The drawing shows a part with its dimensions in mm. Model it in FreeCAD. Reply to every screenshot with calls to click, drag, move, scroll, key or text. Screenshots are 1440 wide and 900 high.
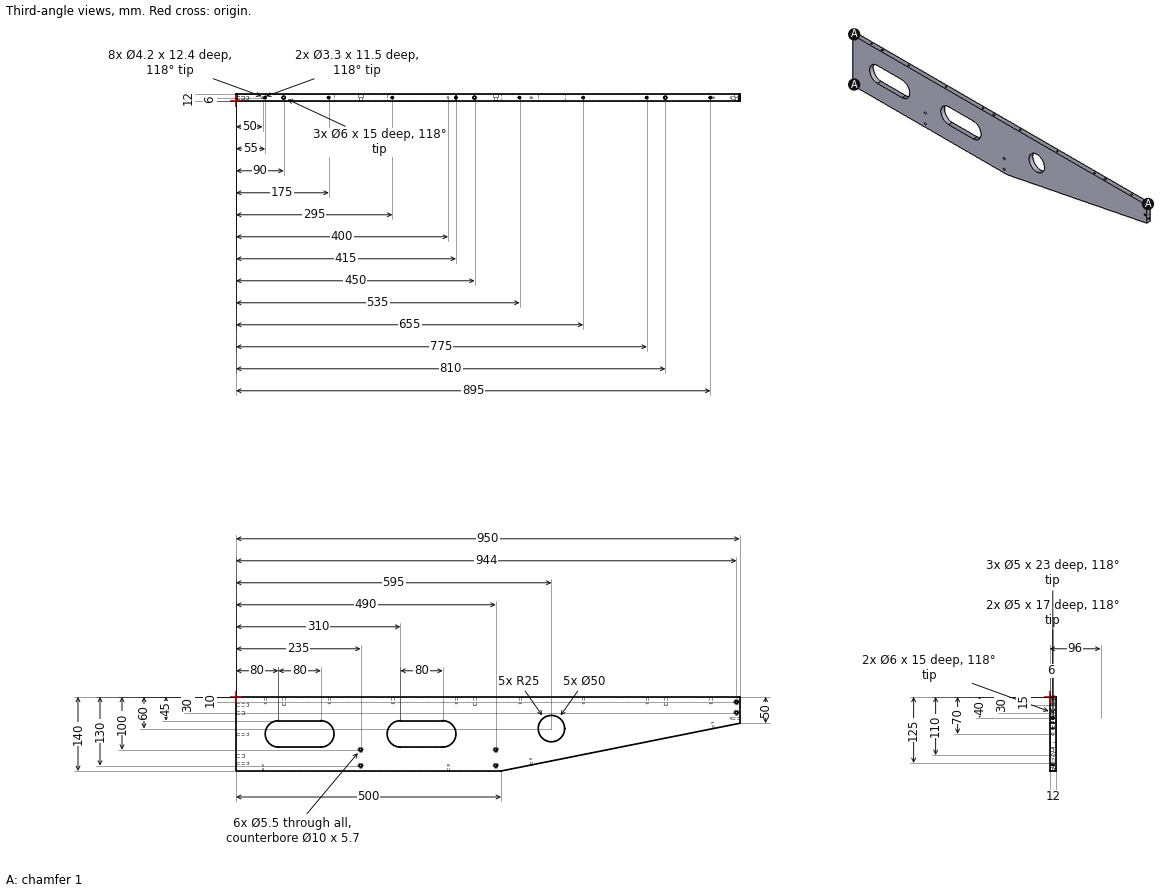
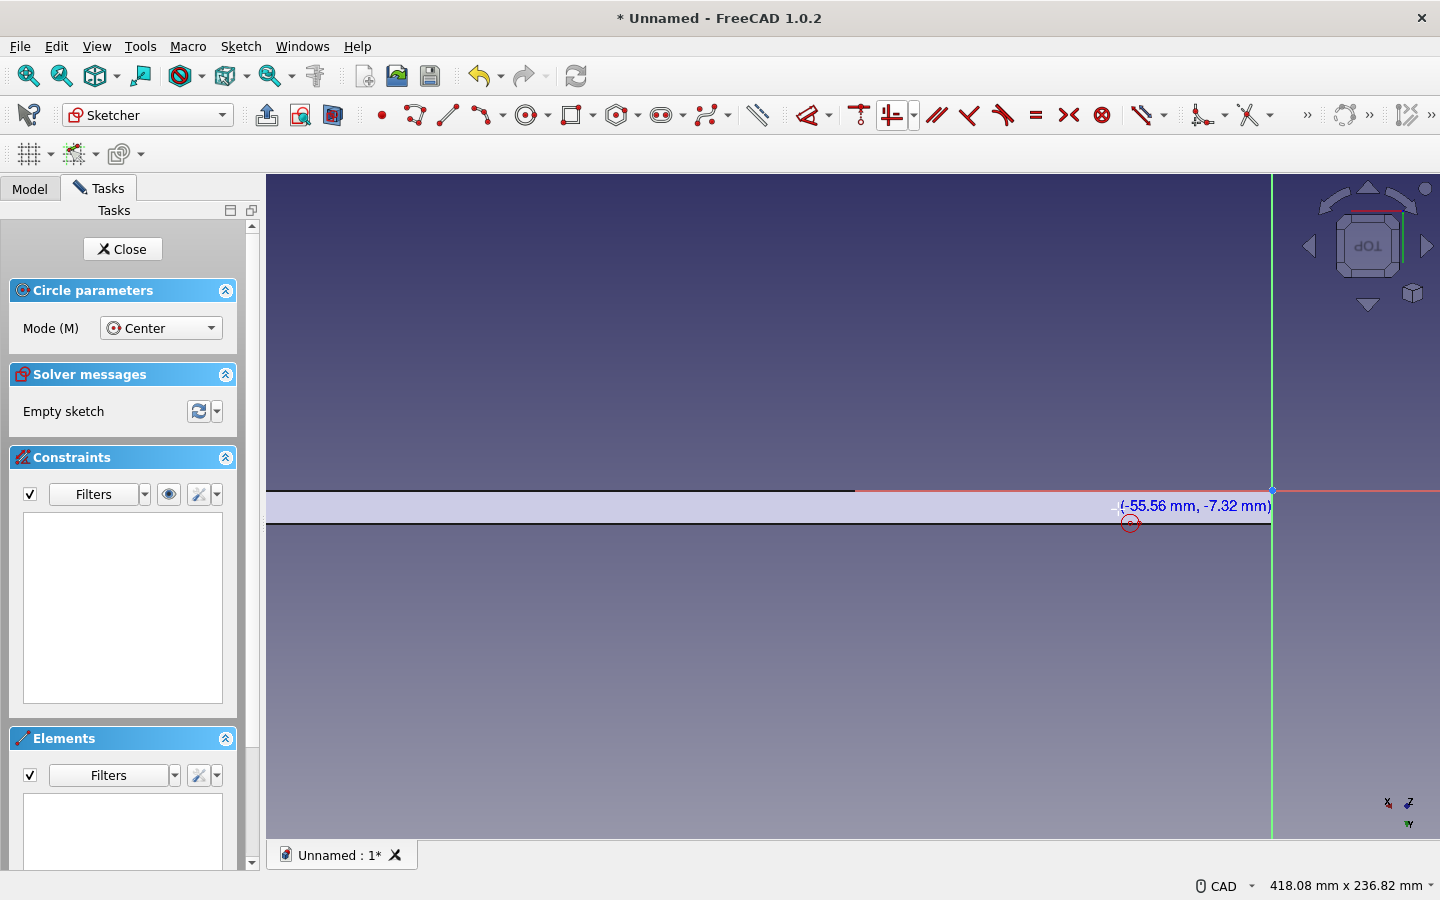
click(1118, 507)
move(1122, 512)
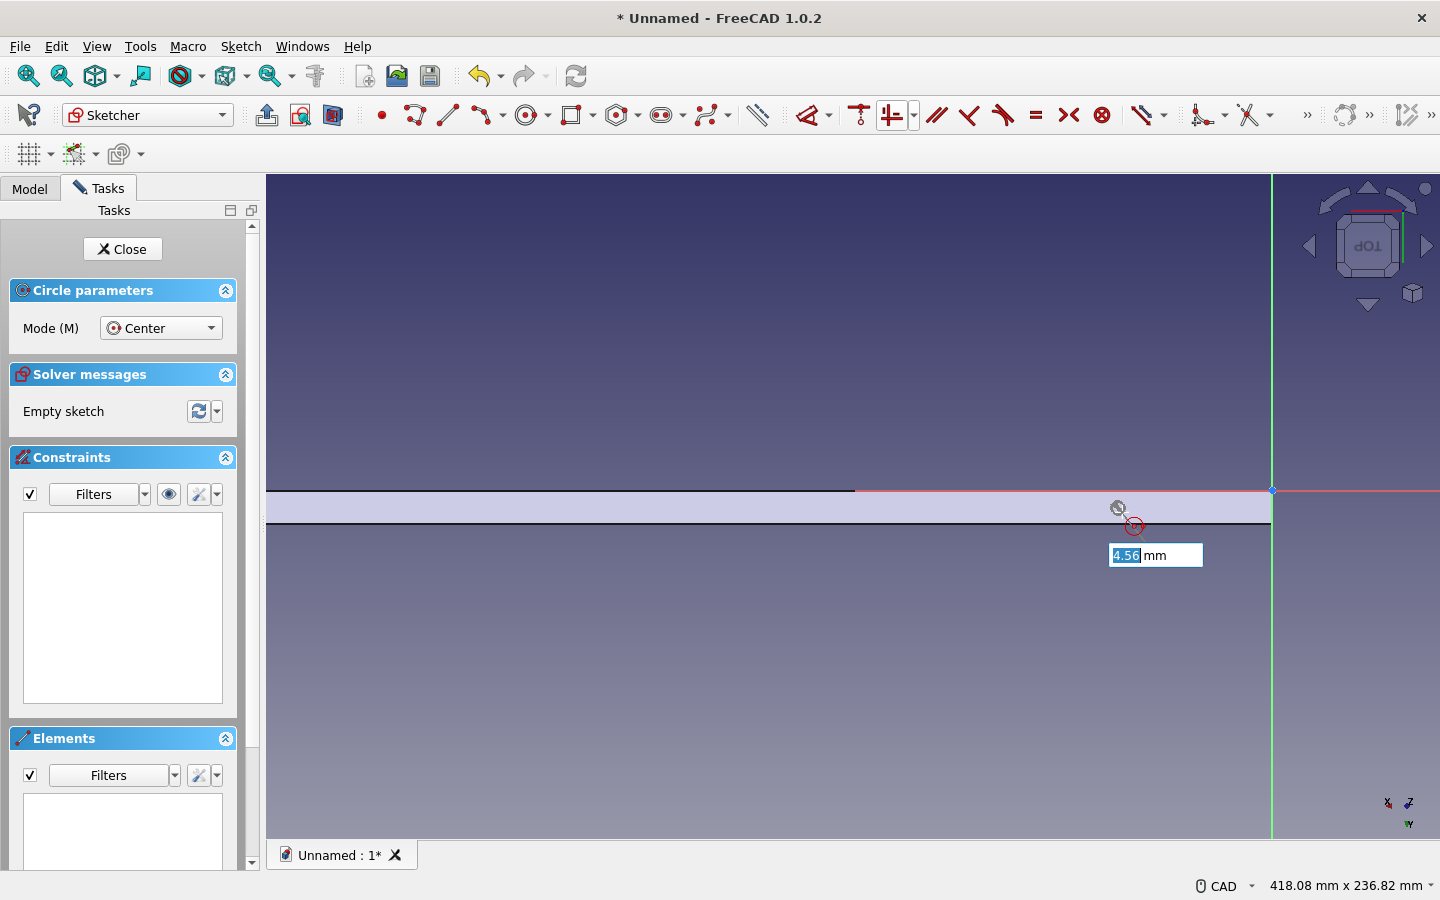
text(4.2)
key(Return)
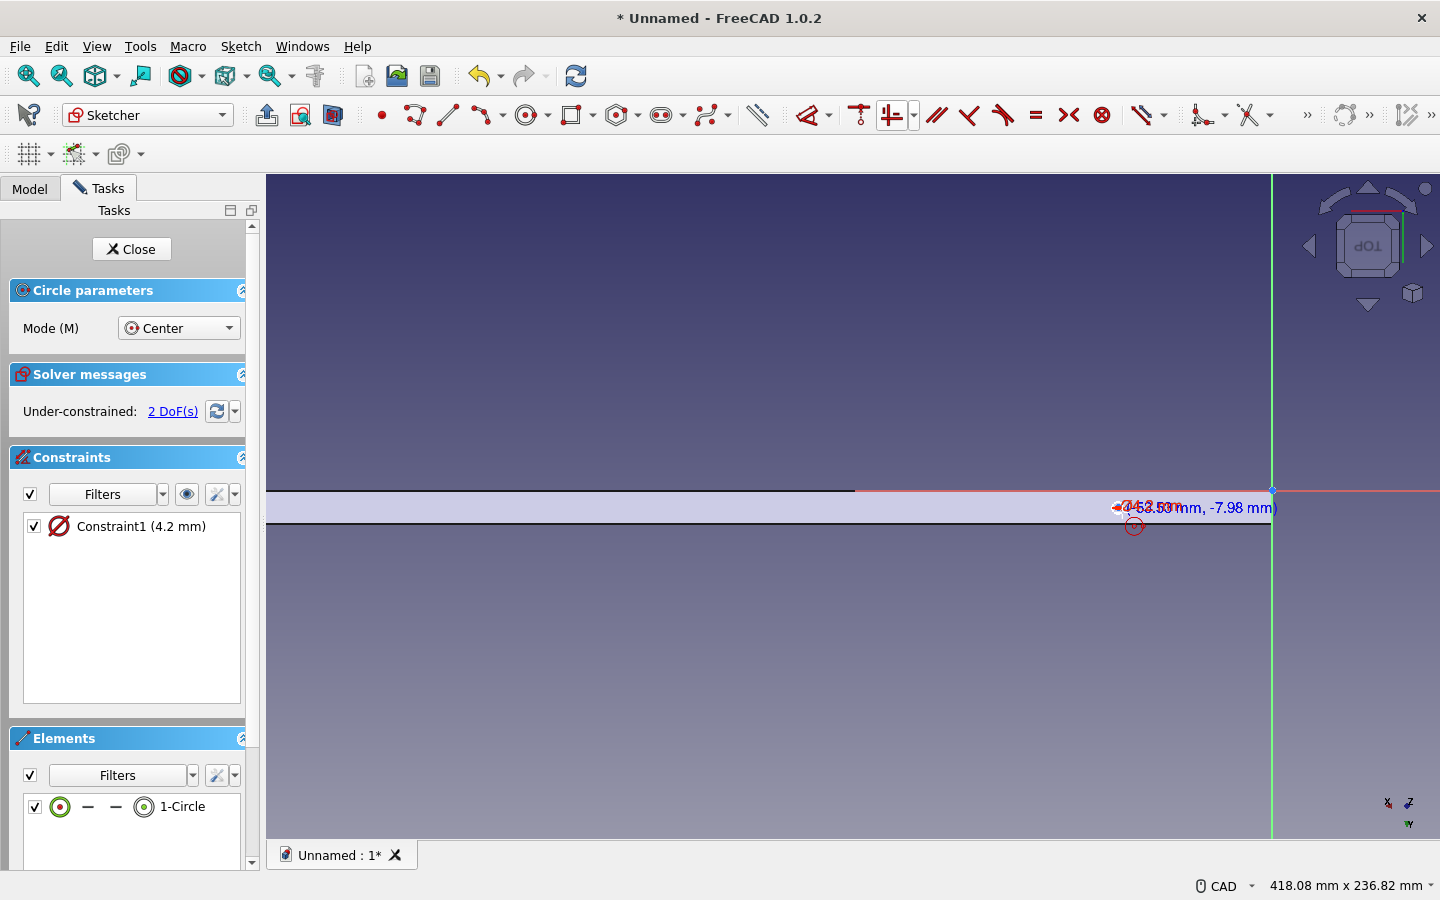
scroll(781, 507, up, 7)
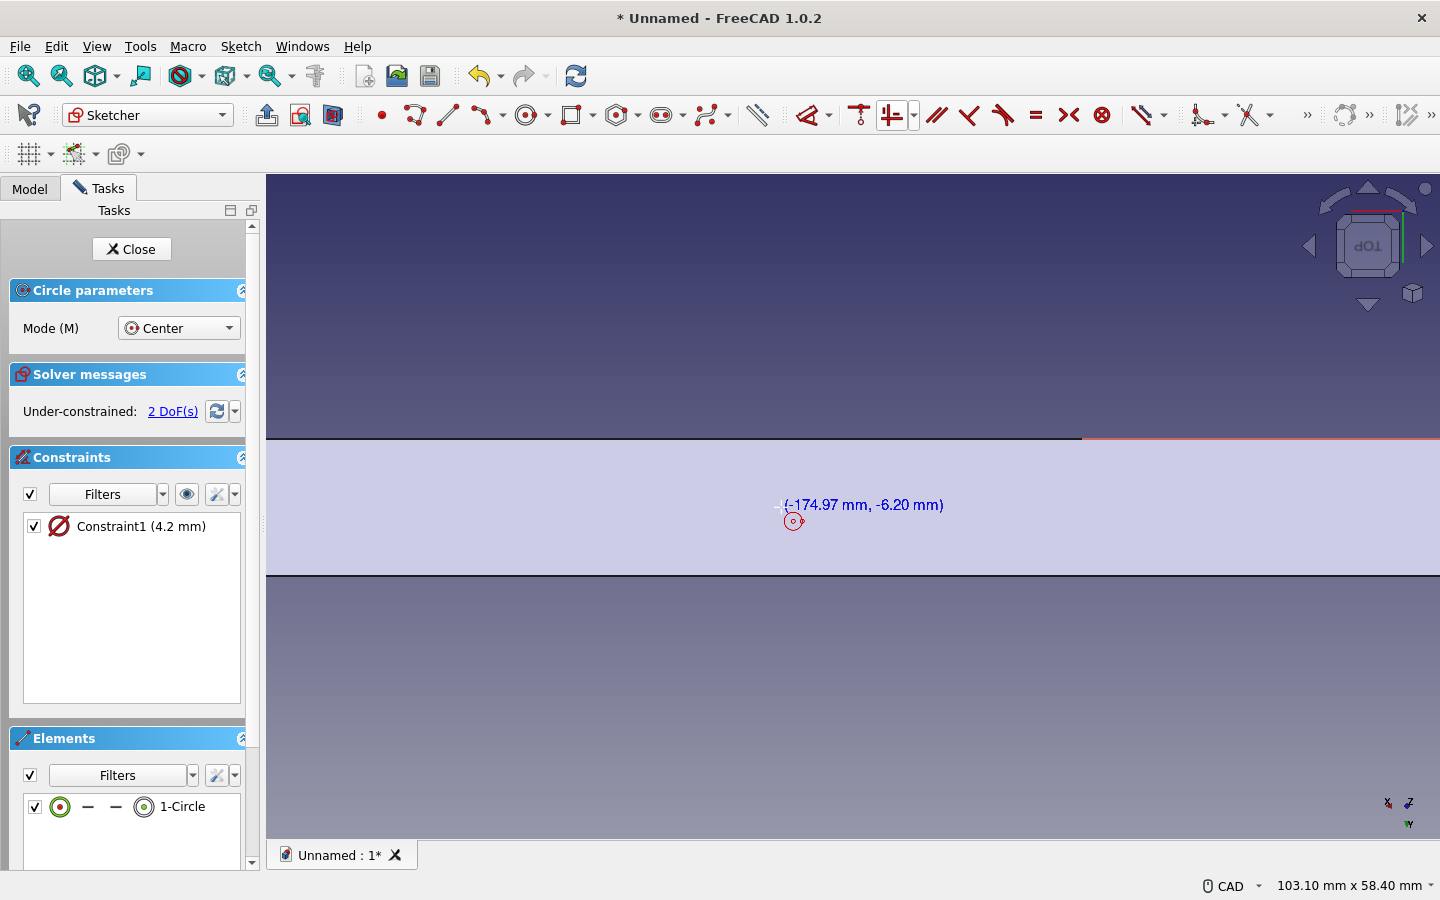
scroll(1035, 508, down, 13)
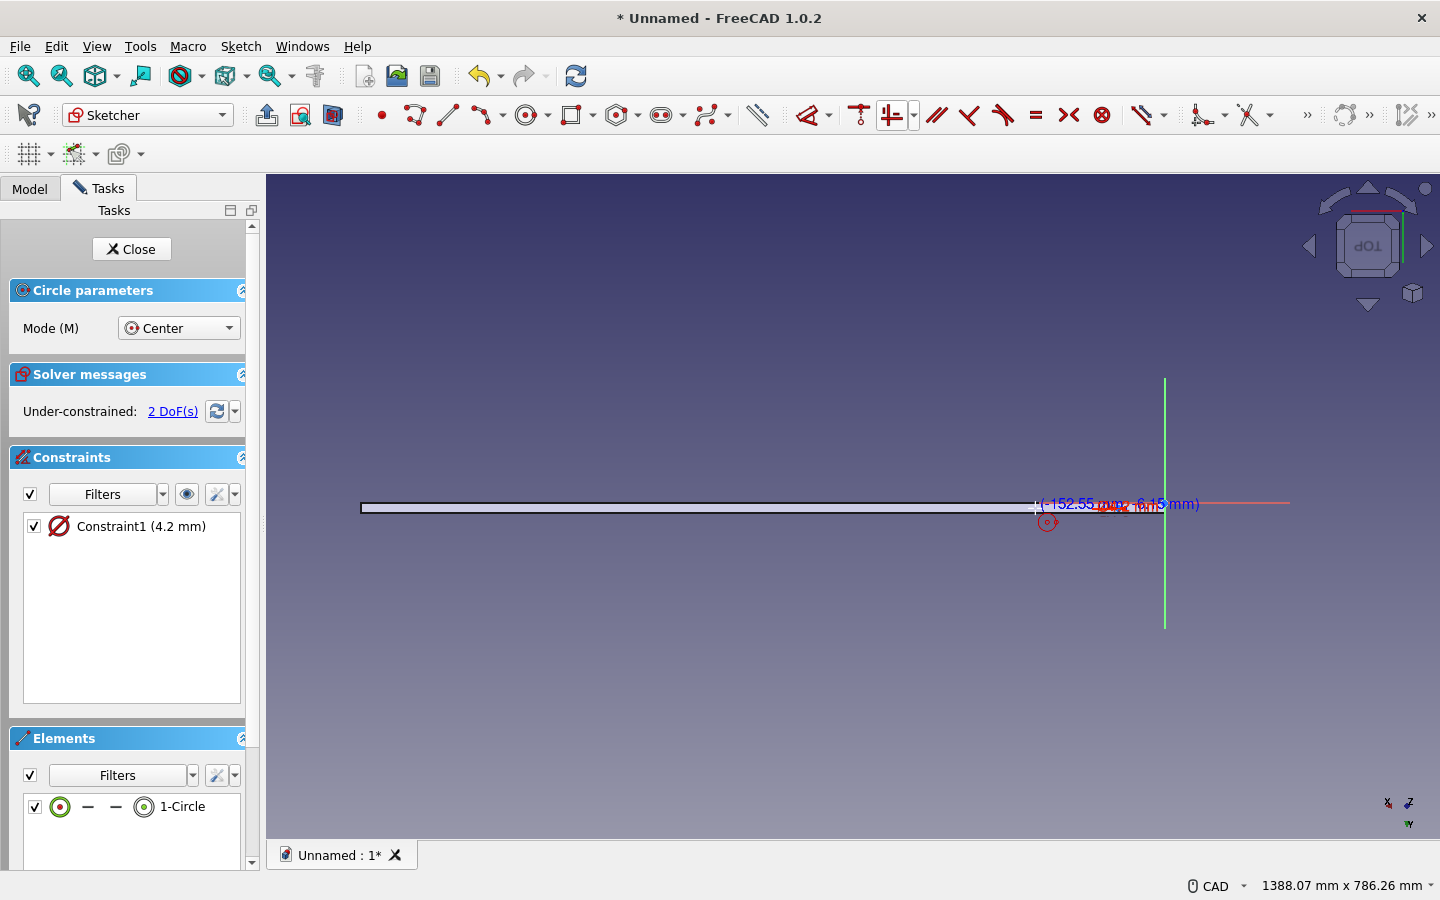
scroll(1017, 508, up, 6)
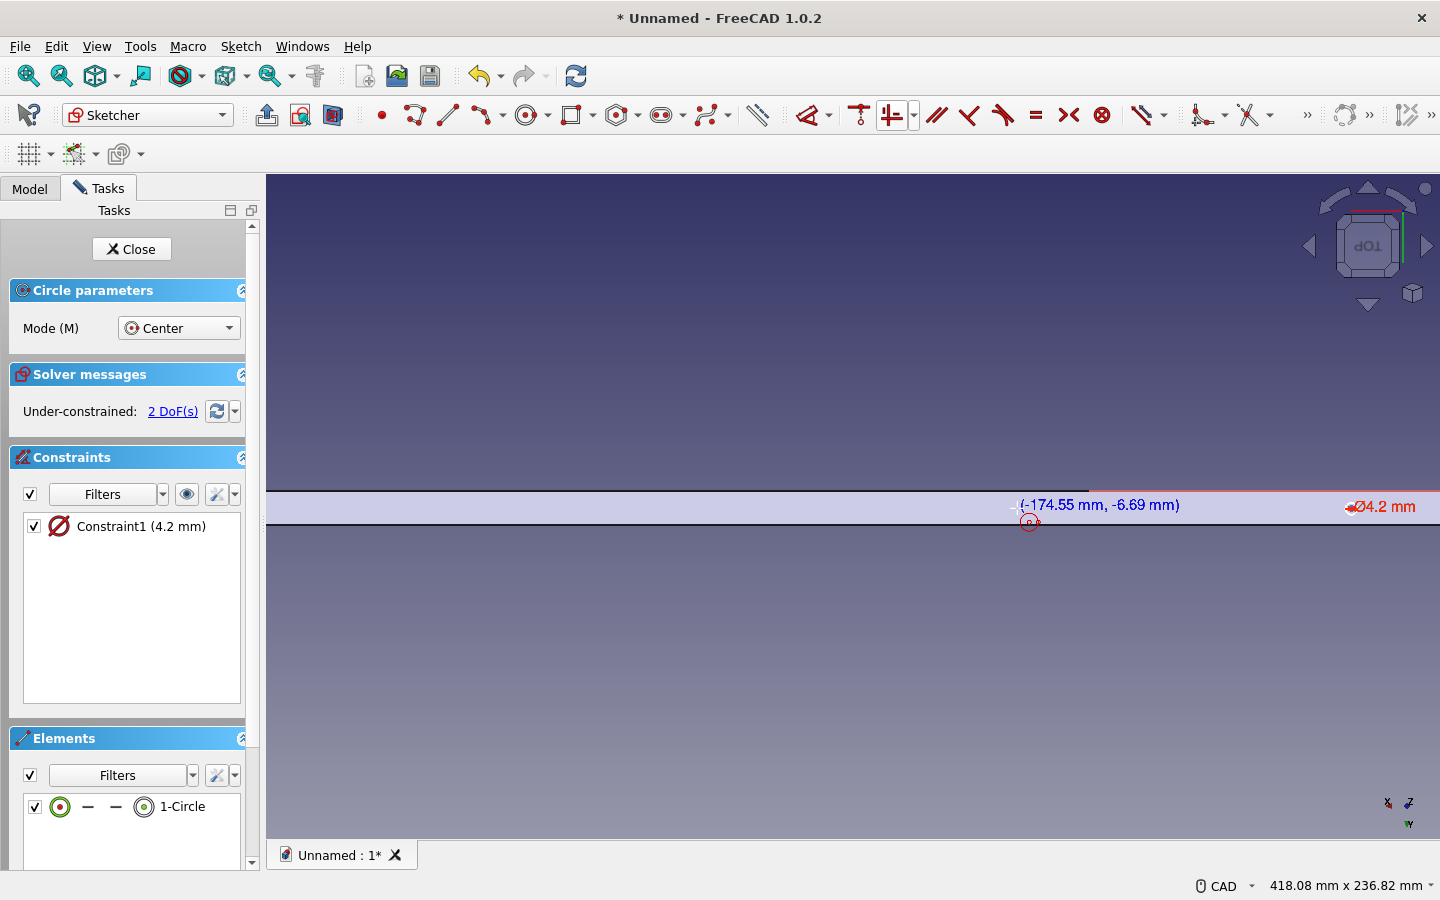
click(1014, 508)
move(1018, 512)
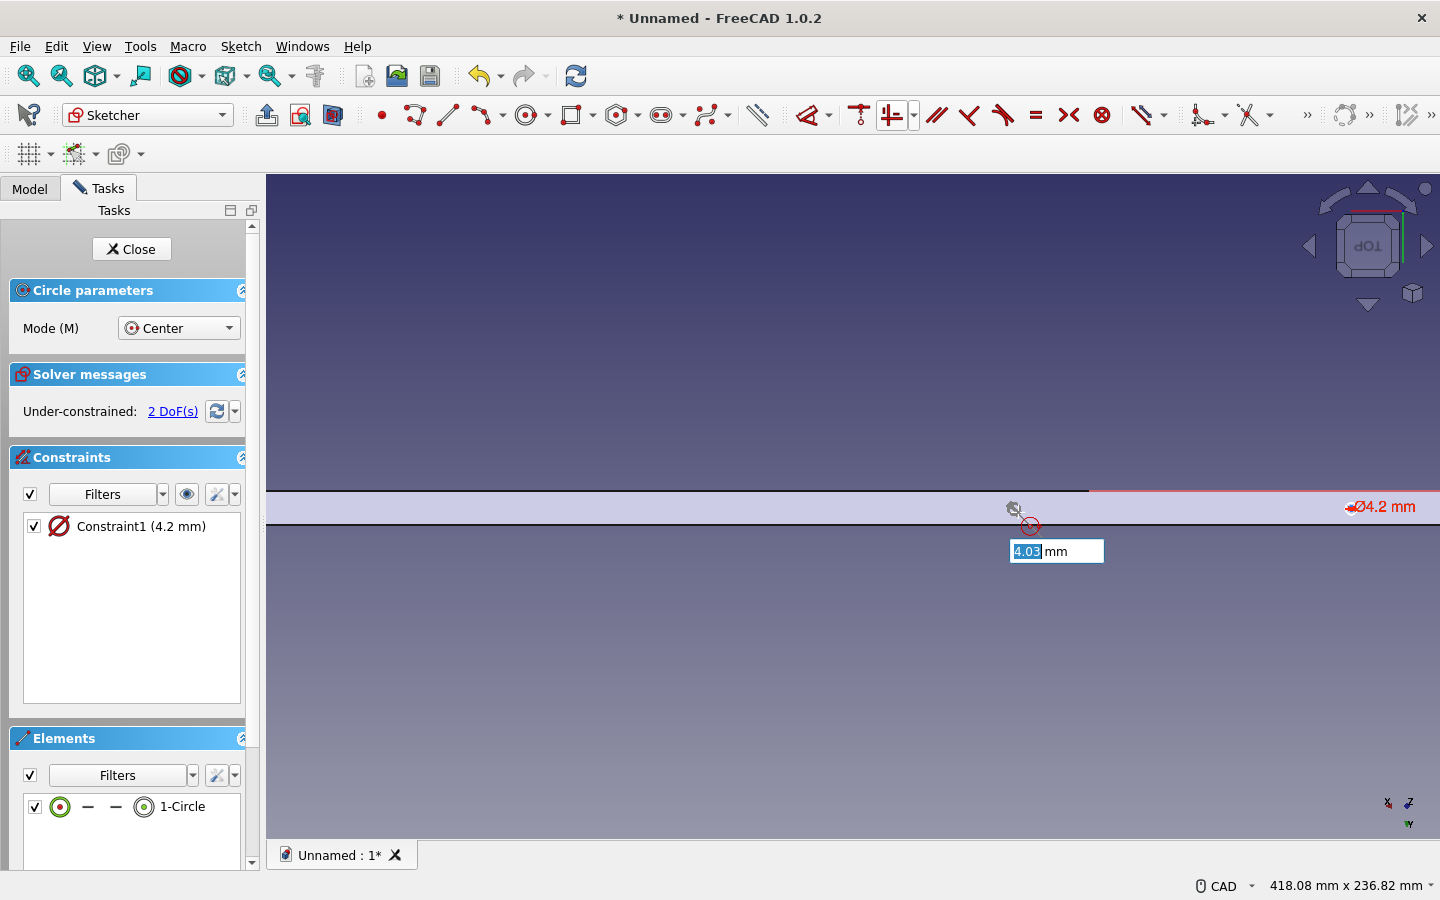
text(4.2)
key(Return)